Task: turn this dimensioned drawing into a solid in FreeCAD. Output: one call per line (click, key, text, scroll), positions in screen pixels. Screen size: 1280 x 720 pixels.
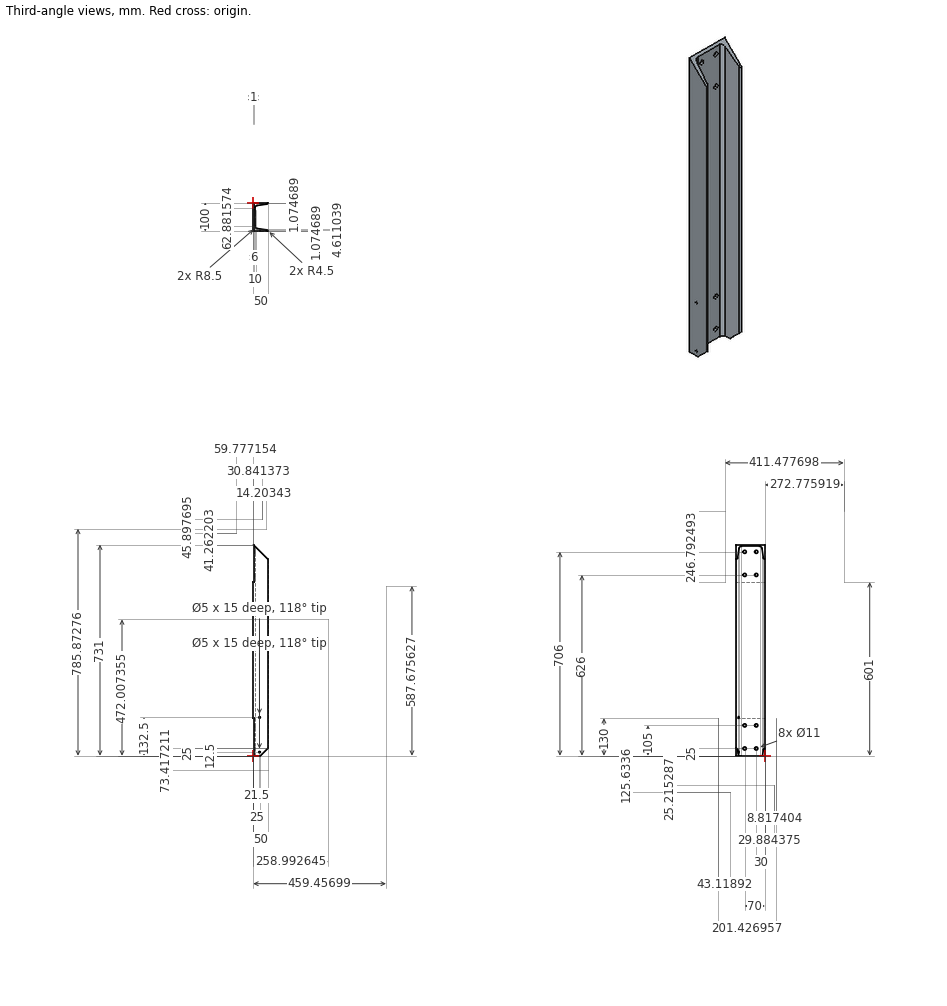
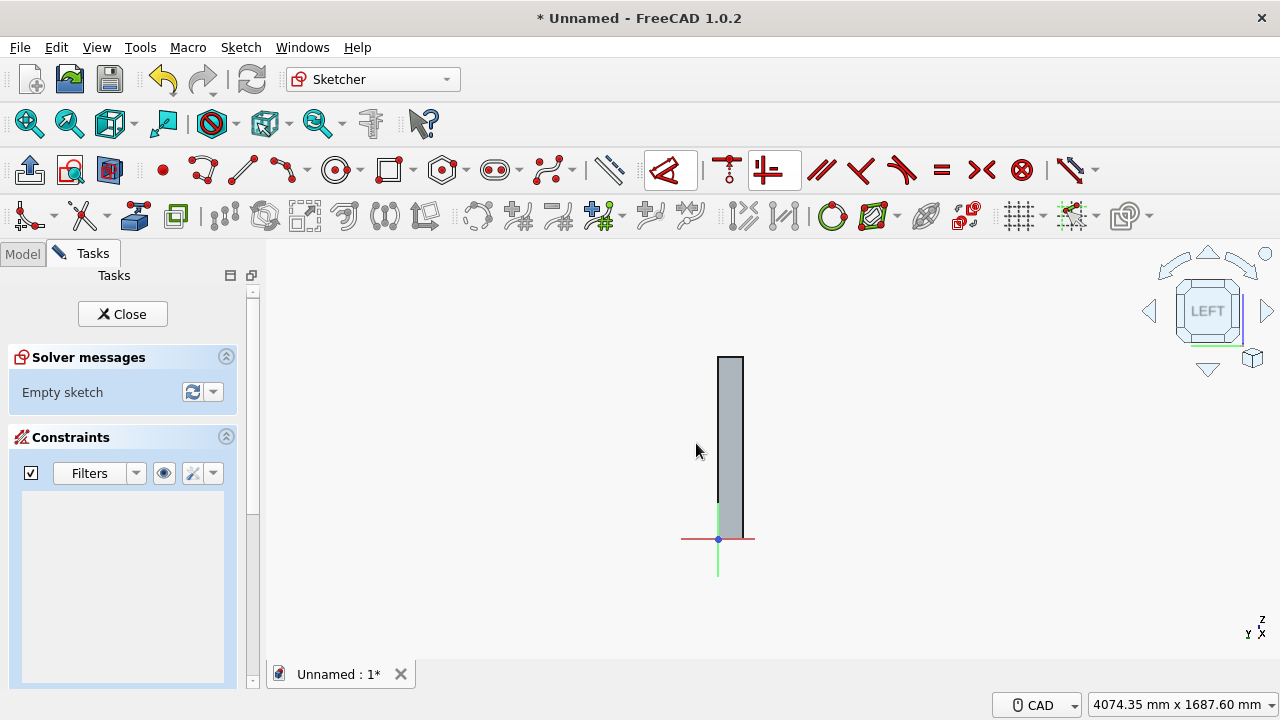
key(g)
key(m)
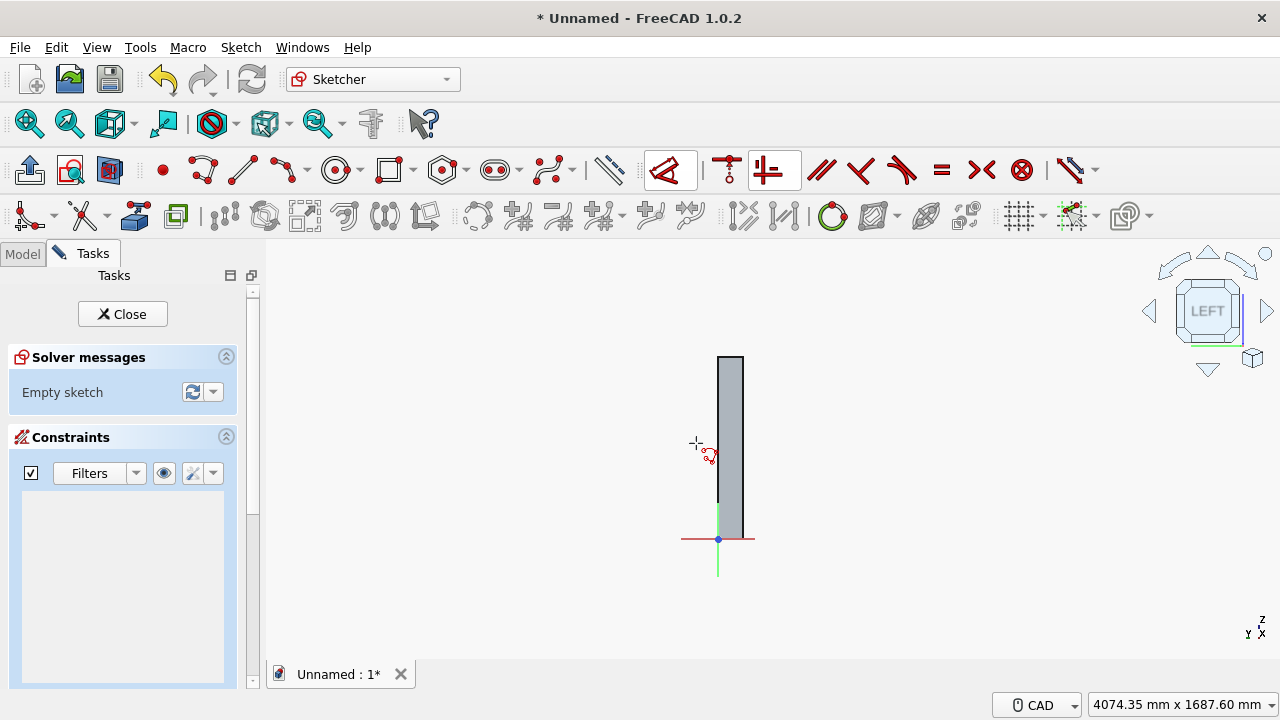
scroll(711, 564, up, 4)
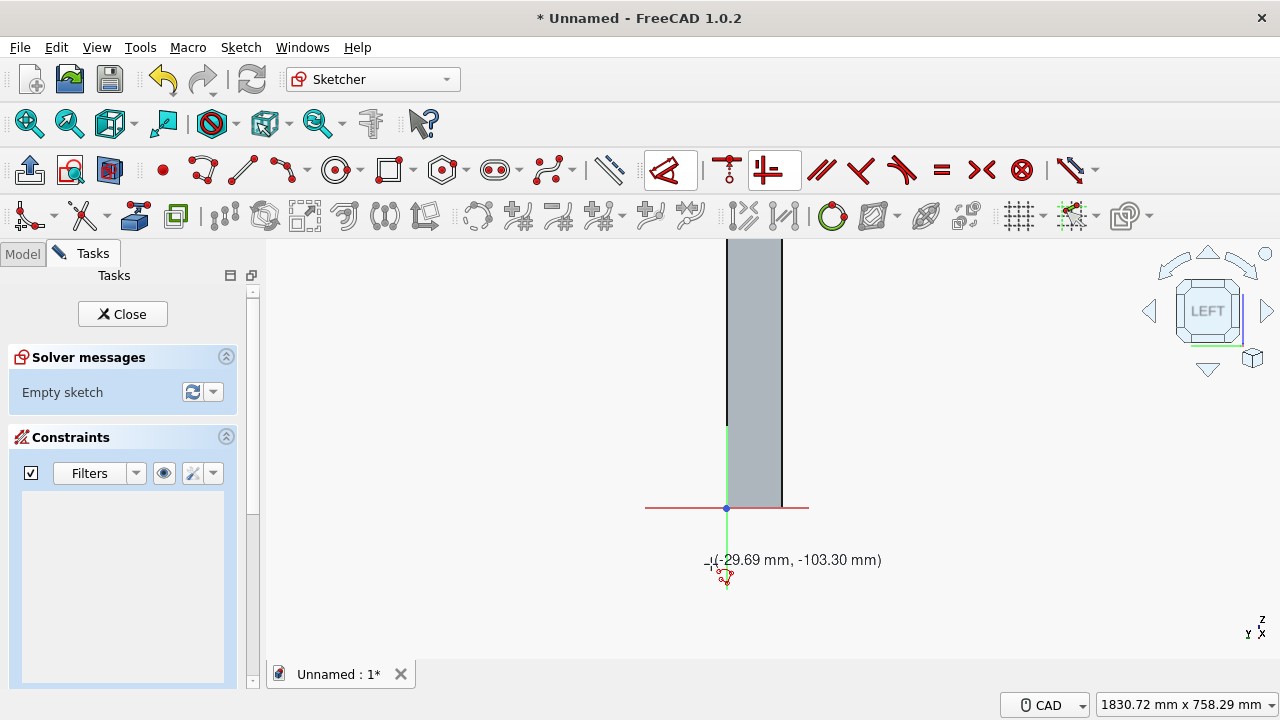
click(710, 564)
click(793, 578)
click(817, 436)
click(705, 436)
click(710, 565)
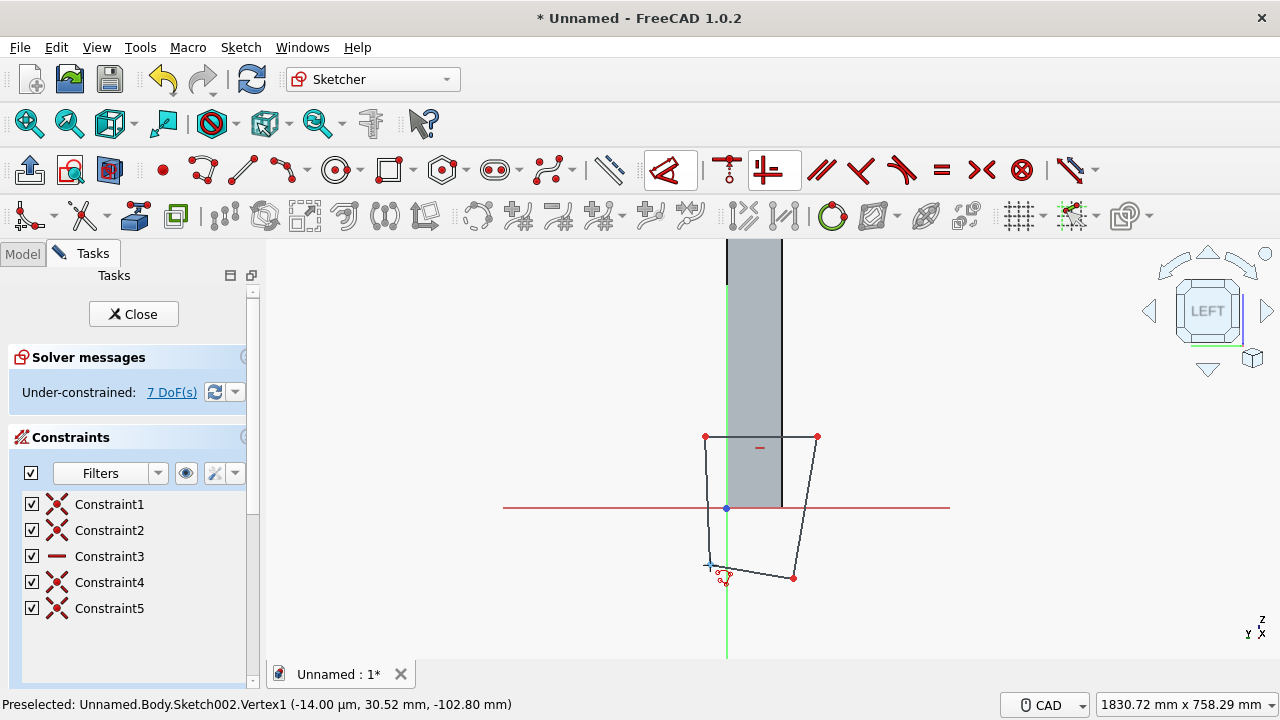
click(390, 170)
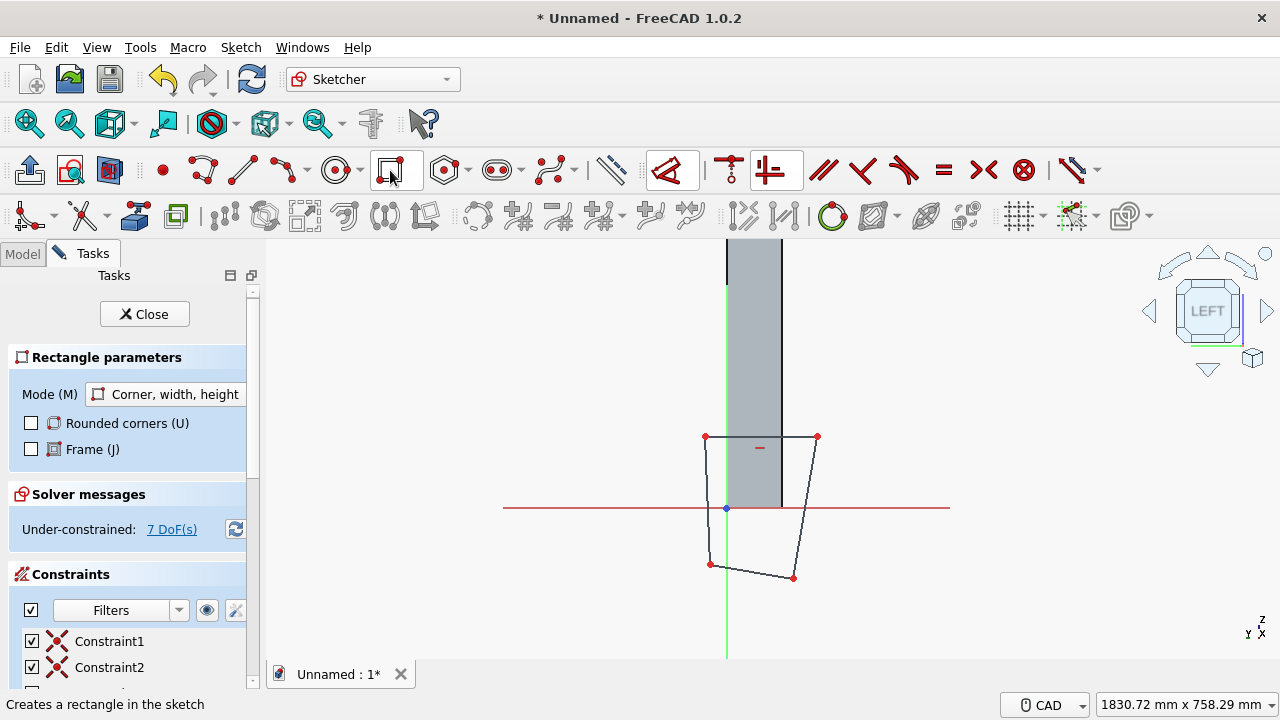
scroll(711, 564, down, 4)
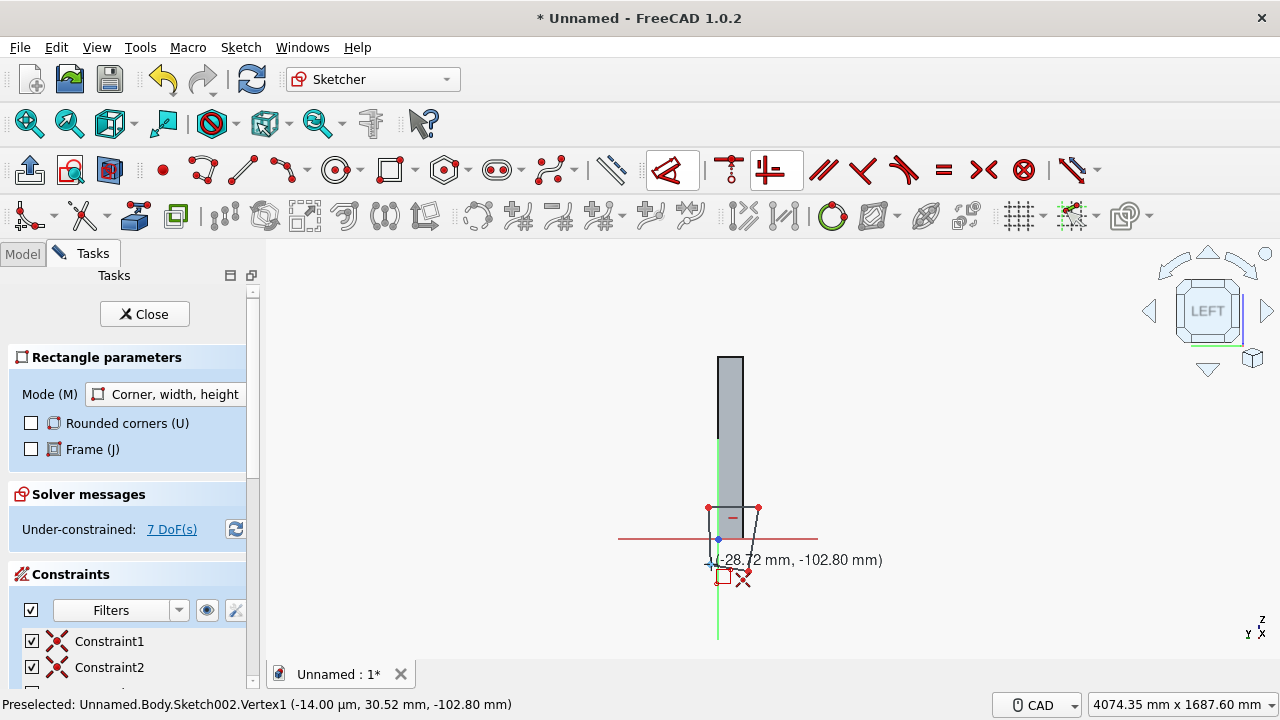
click(651, 328)
move(753, 390)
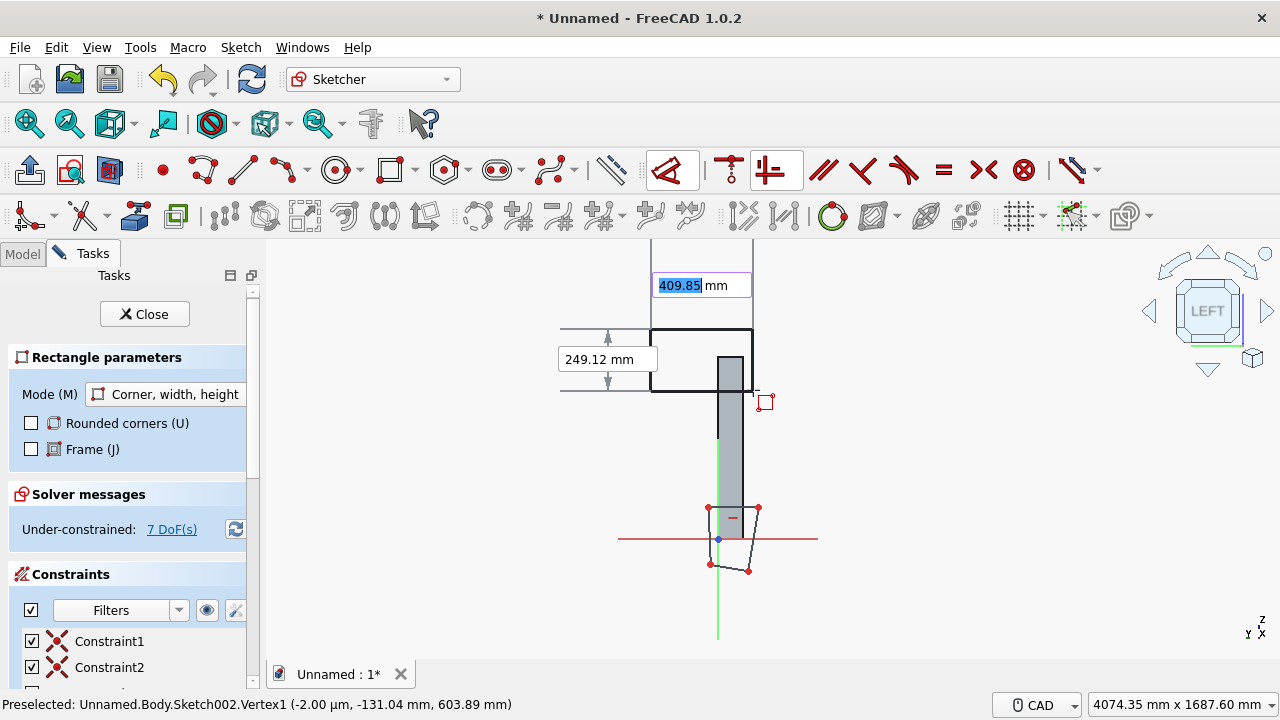
text(411.477698)
key(Tab)
text(246.792493)
key(Return)
key(Escape)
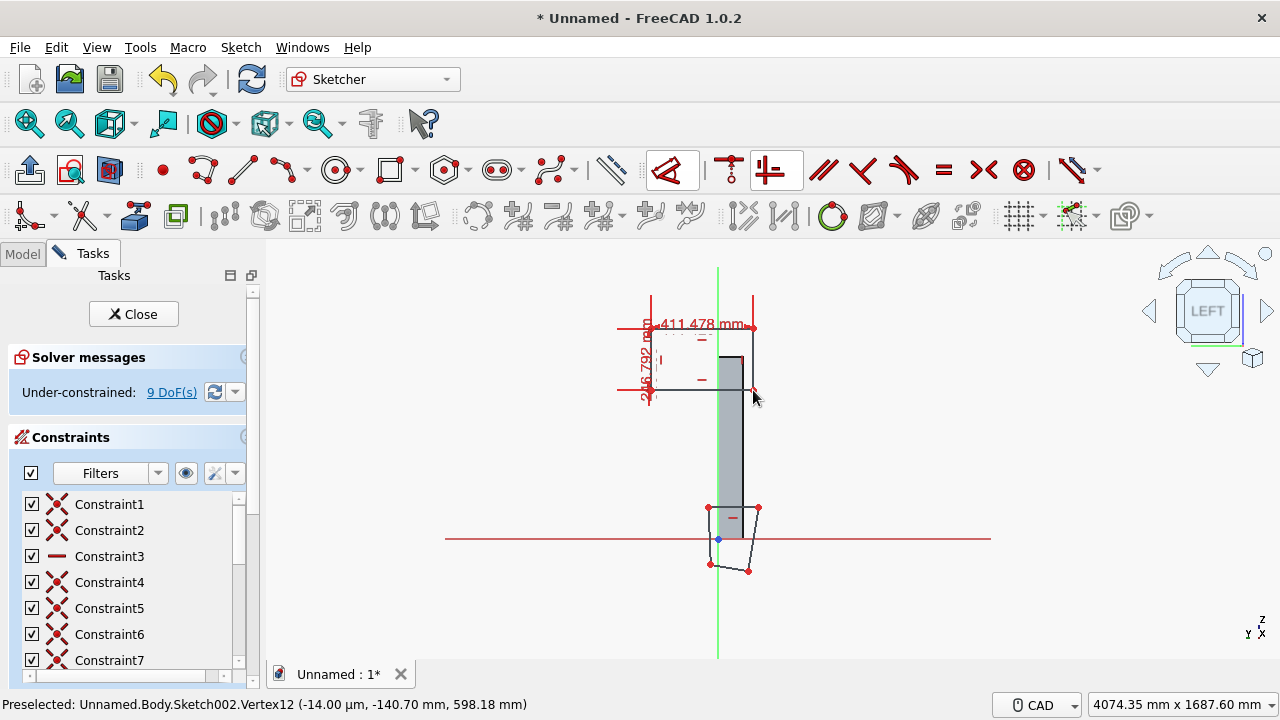
scroll(759, 507, up, 2)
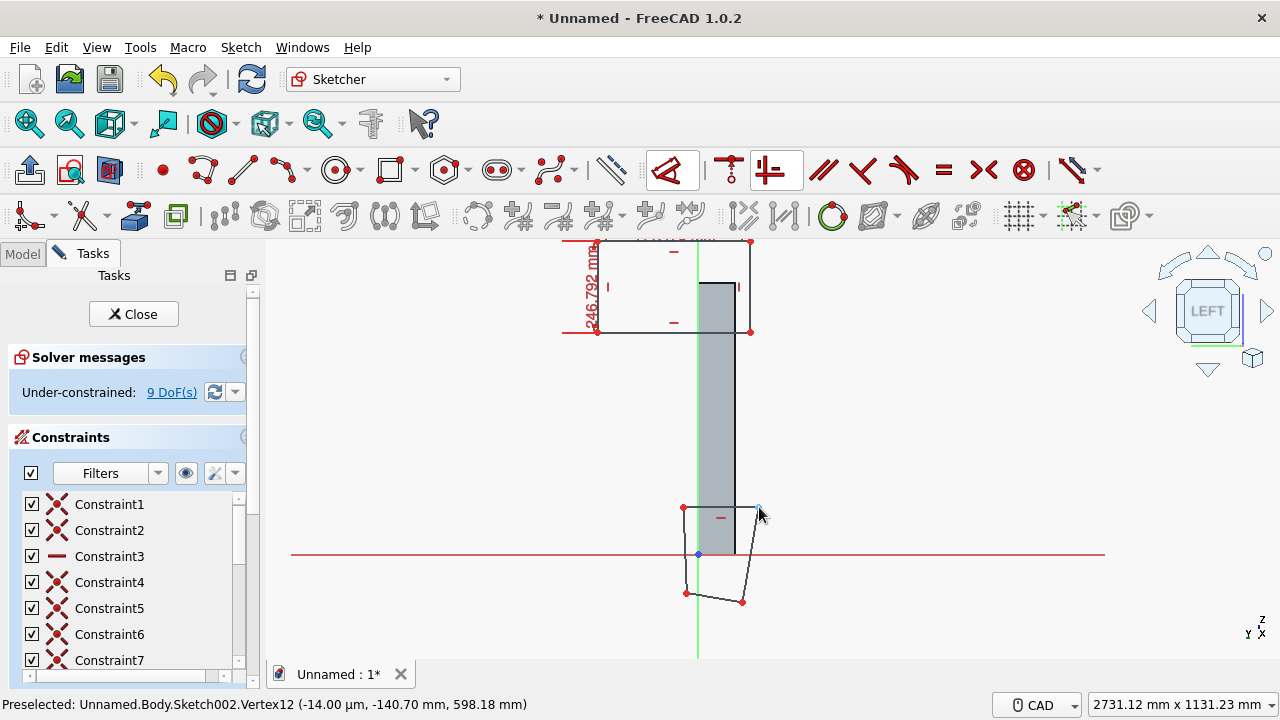
click(759, 507)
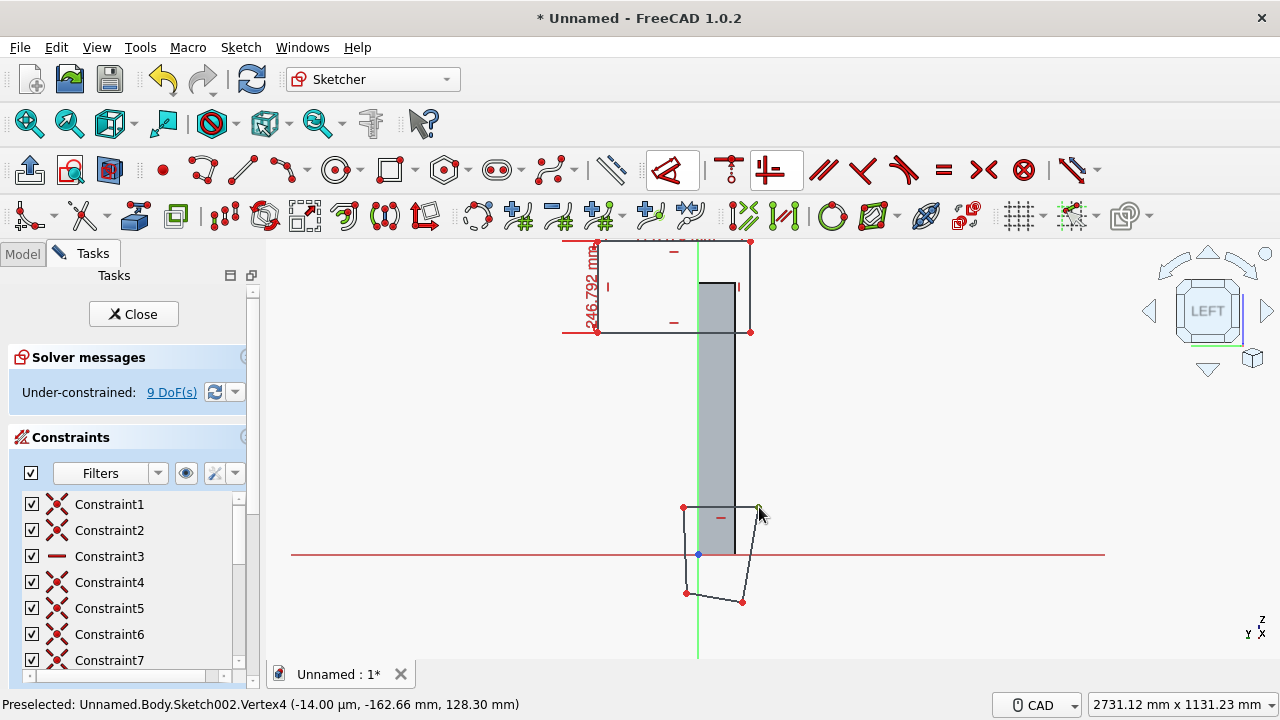
click(694, 170)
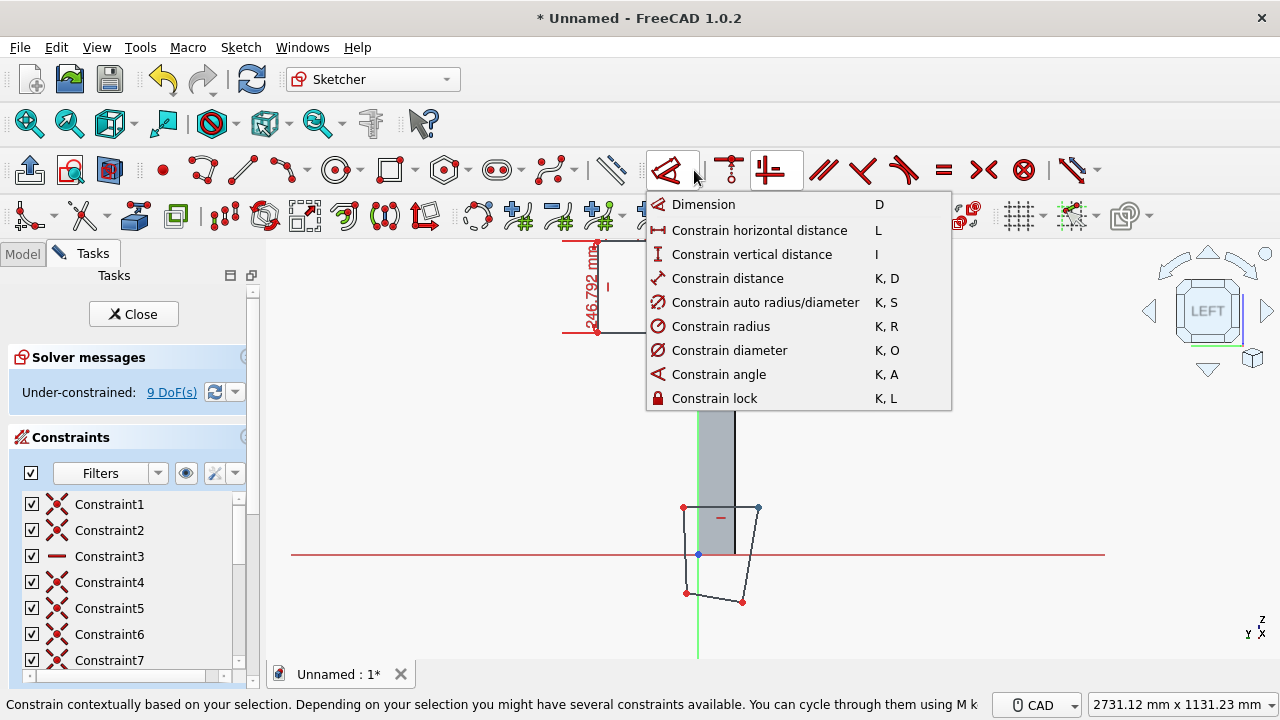
click(799, 254)